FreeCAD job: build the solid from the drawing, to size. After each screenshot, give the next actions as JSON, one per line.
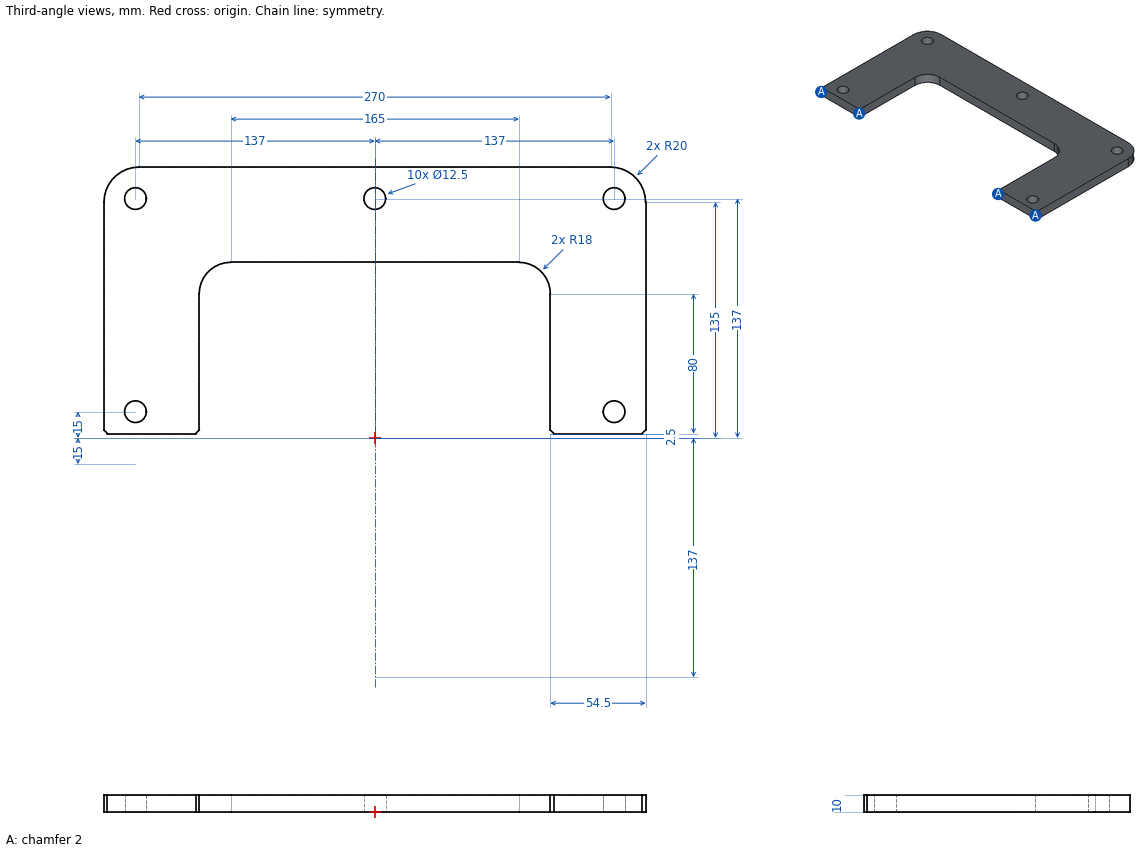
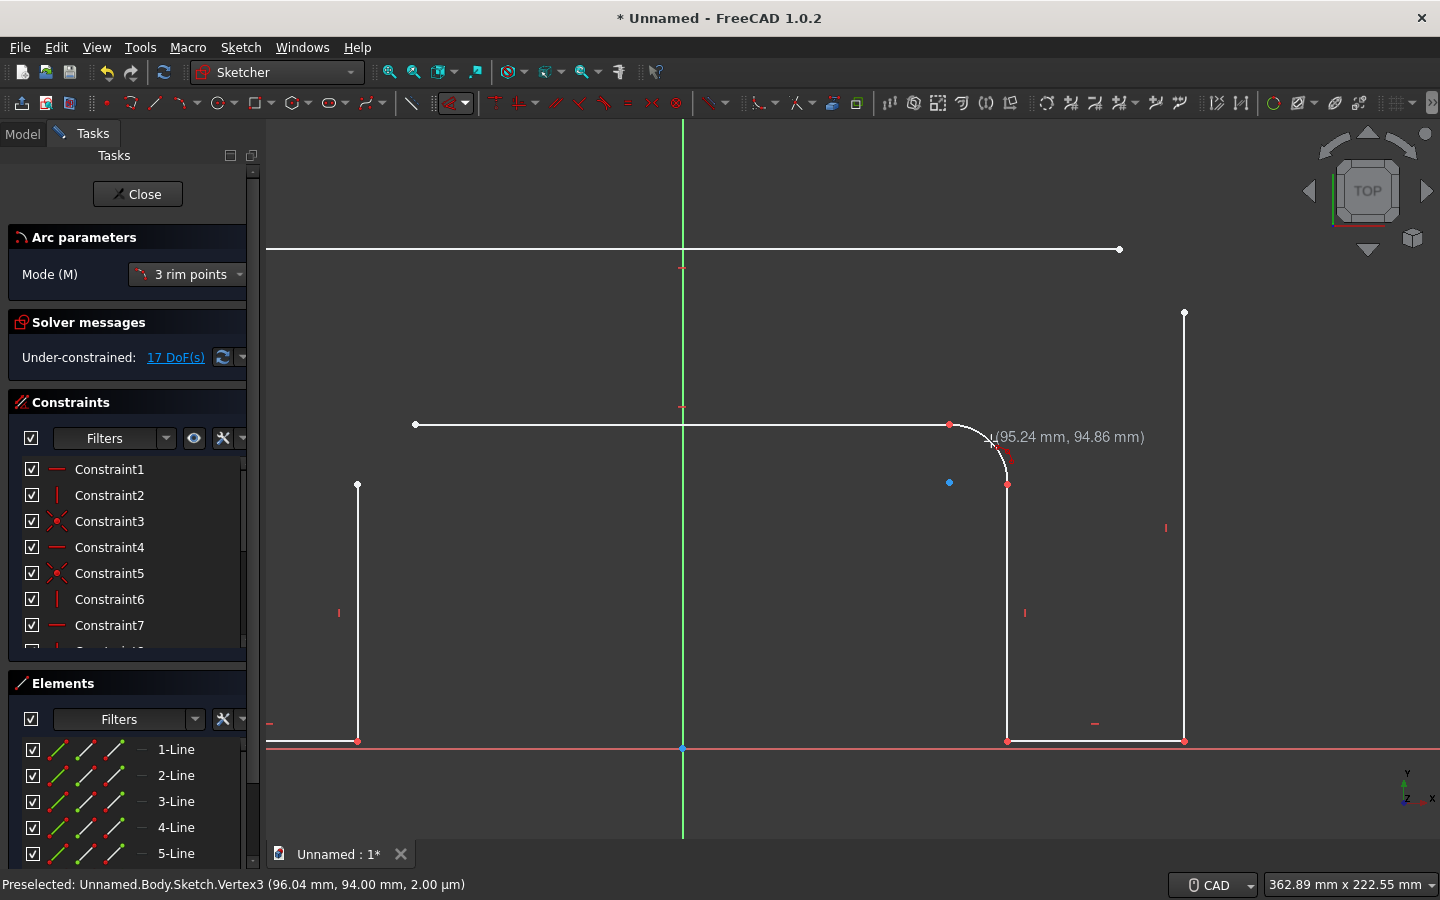
{"action": "left_click", "coordinate": [1184, 313]}
{"action": "left_click", "coordinate": [1119, 249]}
{"action": "left_click", "coordinate": [1165, 266]}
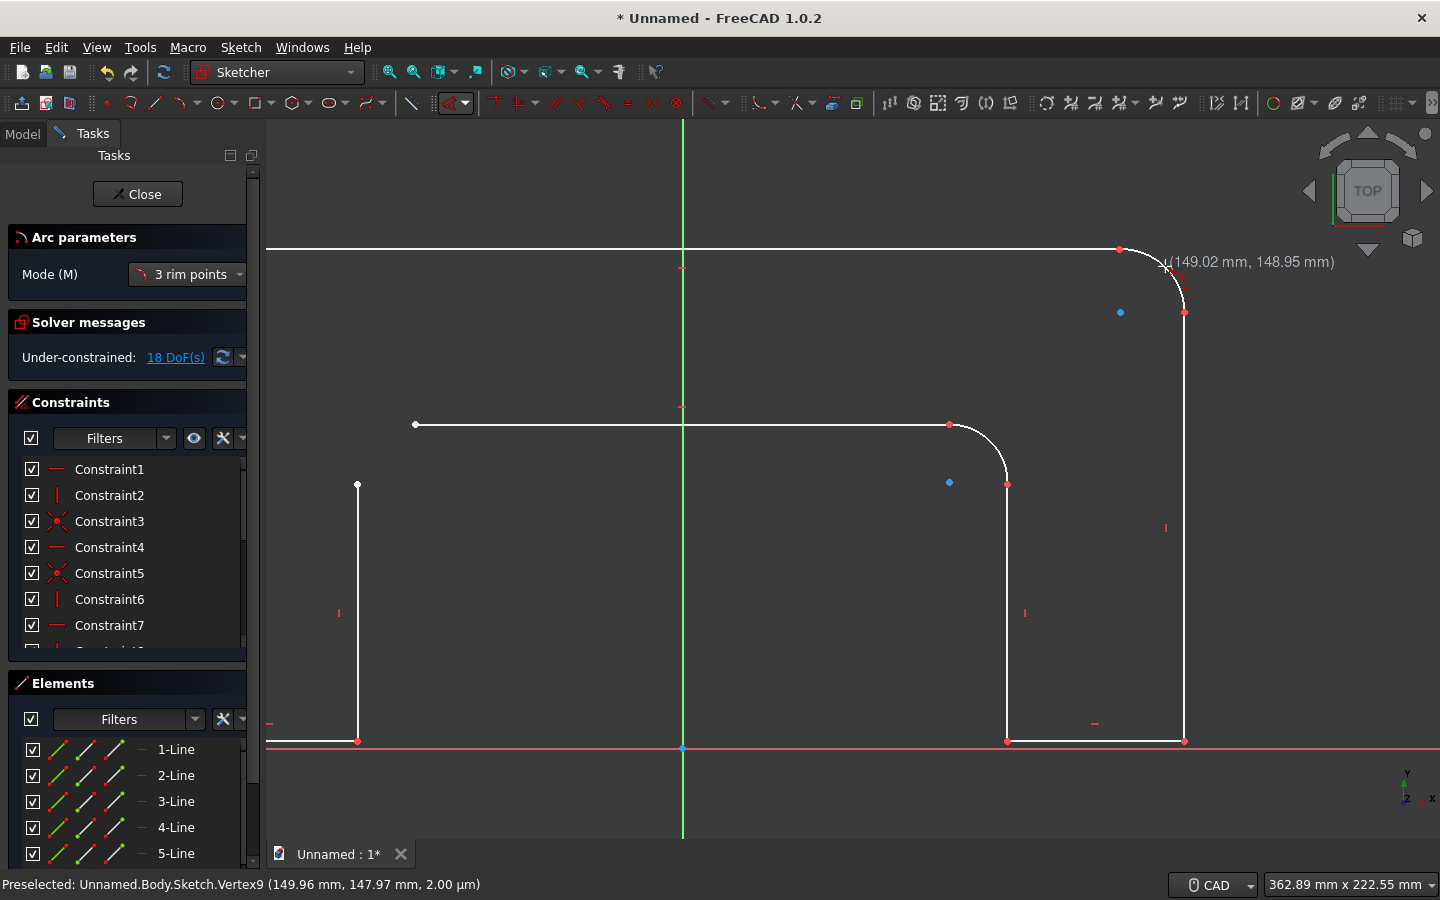
{"action": "scroll", "coordinate": [991, 440], "scroll_direction": "down", "scroll_amount": 2}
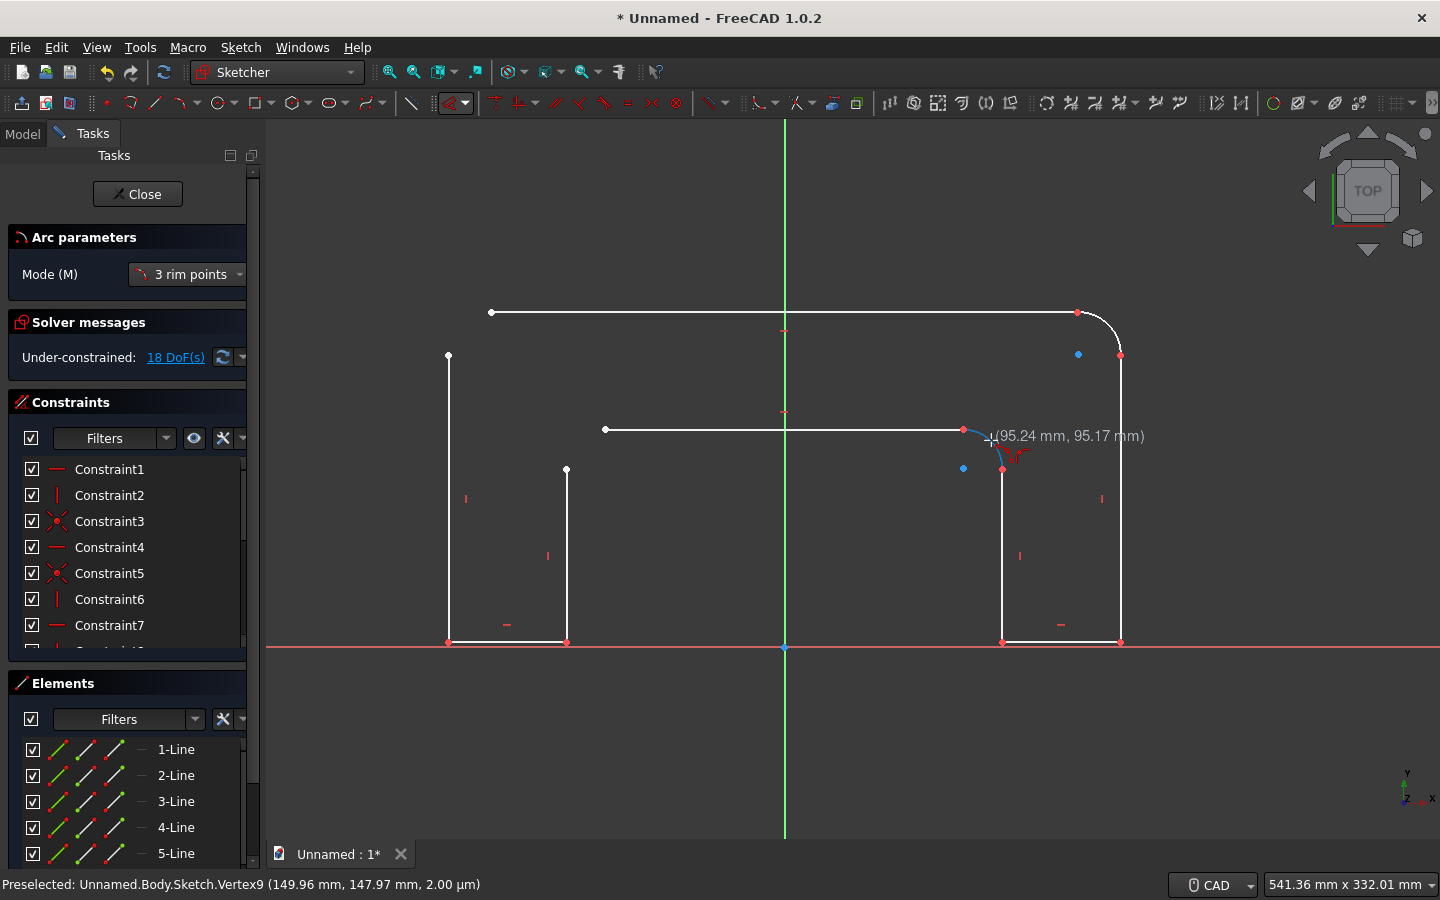
{"action": "left_click", "coordinate": [492, 312]}
{"action": "left_click", "coordinate": [449, 355]}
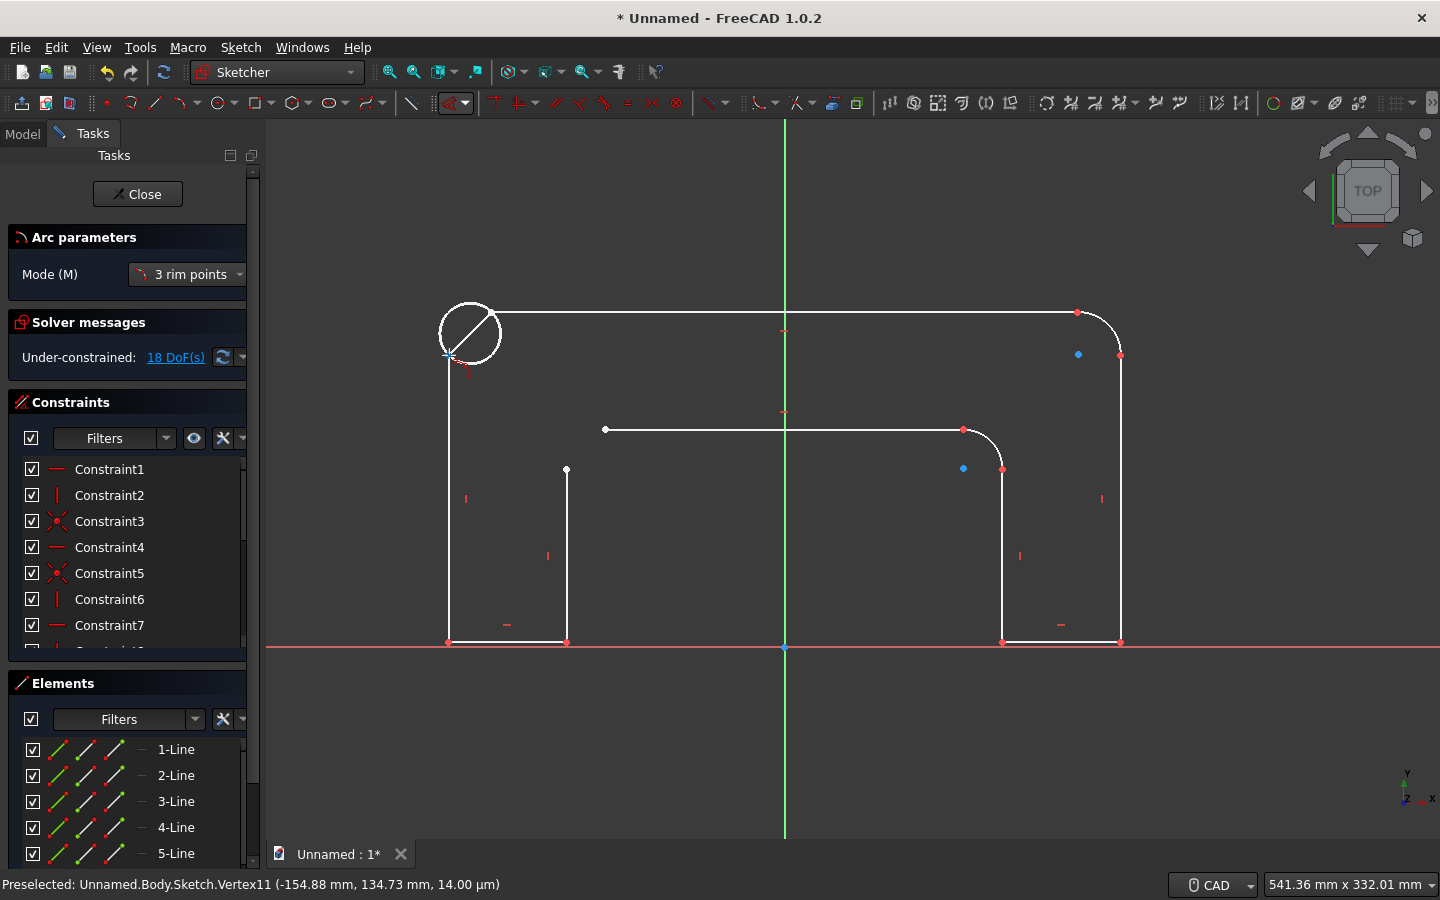
{"action": "scroll", "coordinate": [461, 324], "scroll_direction": "up", "scroll_amount": 2}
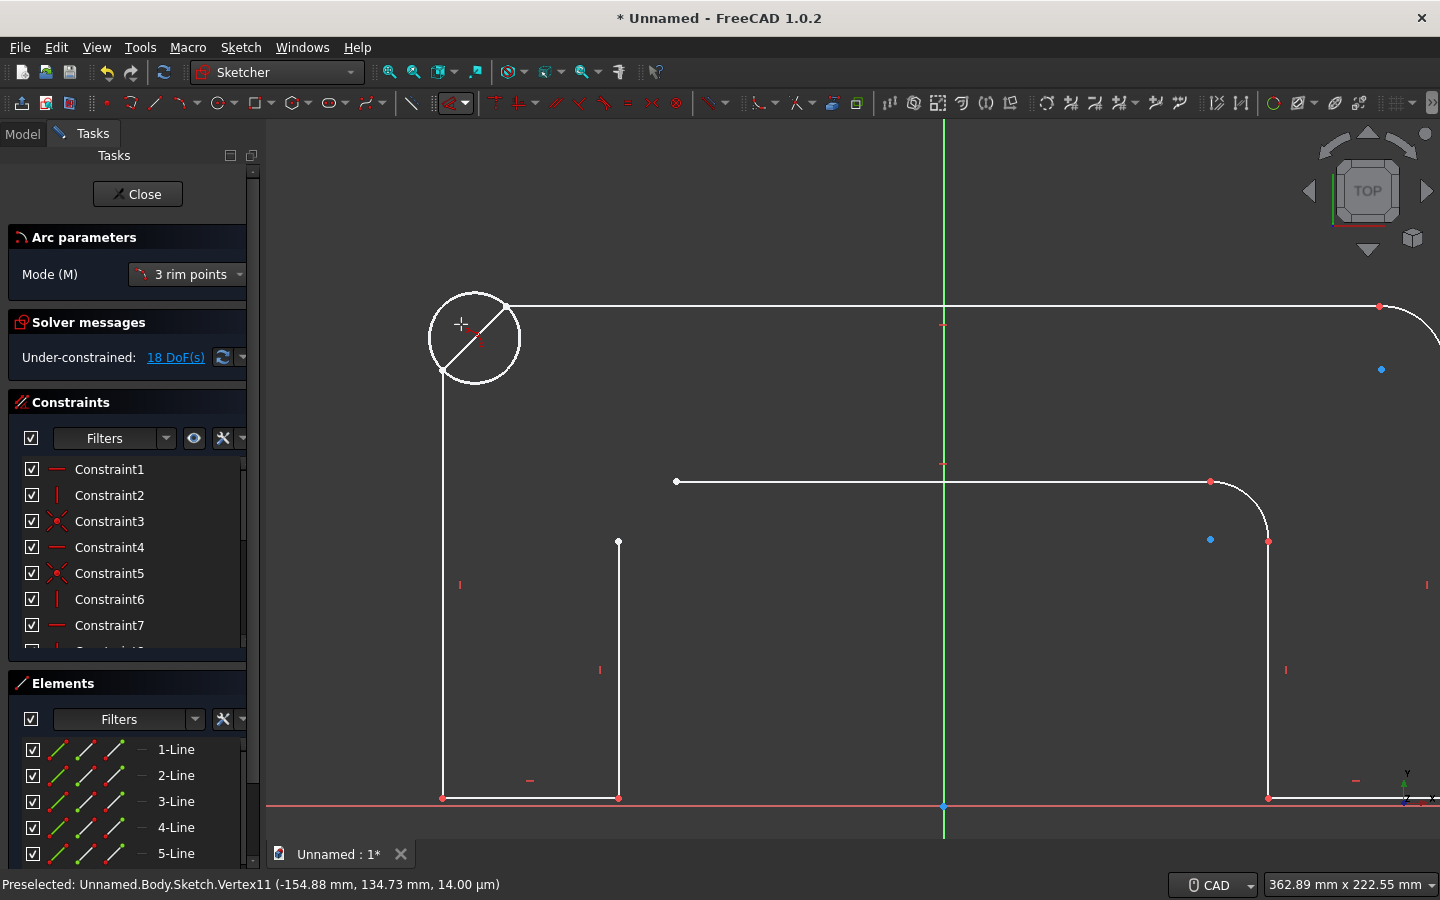
{"action": "left_click", "coordinate": [461, 324]}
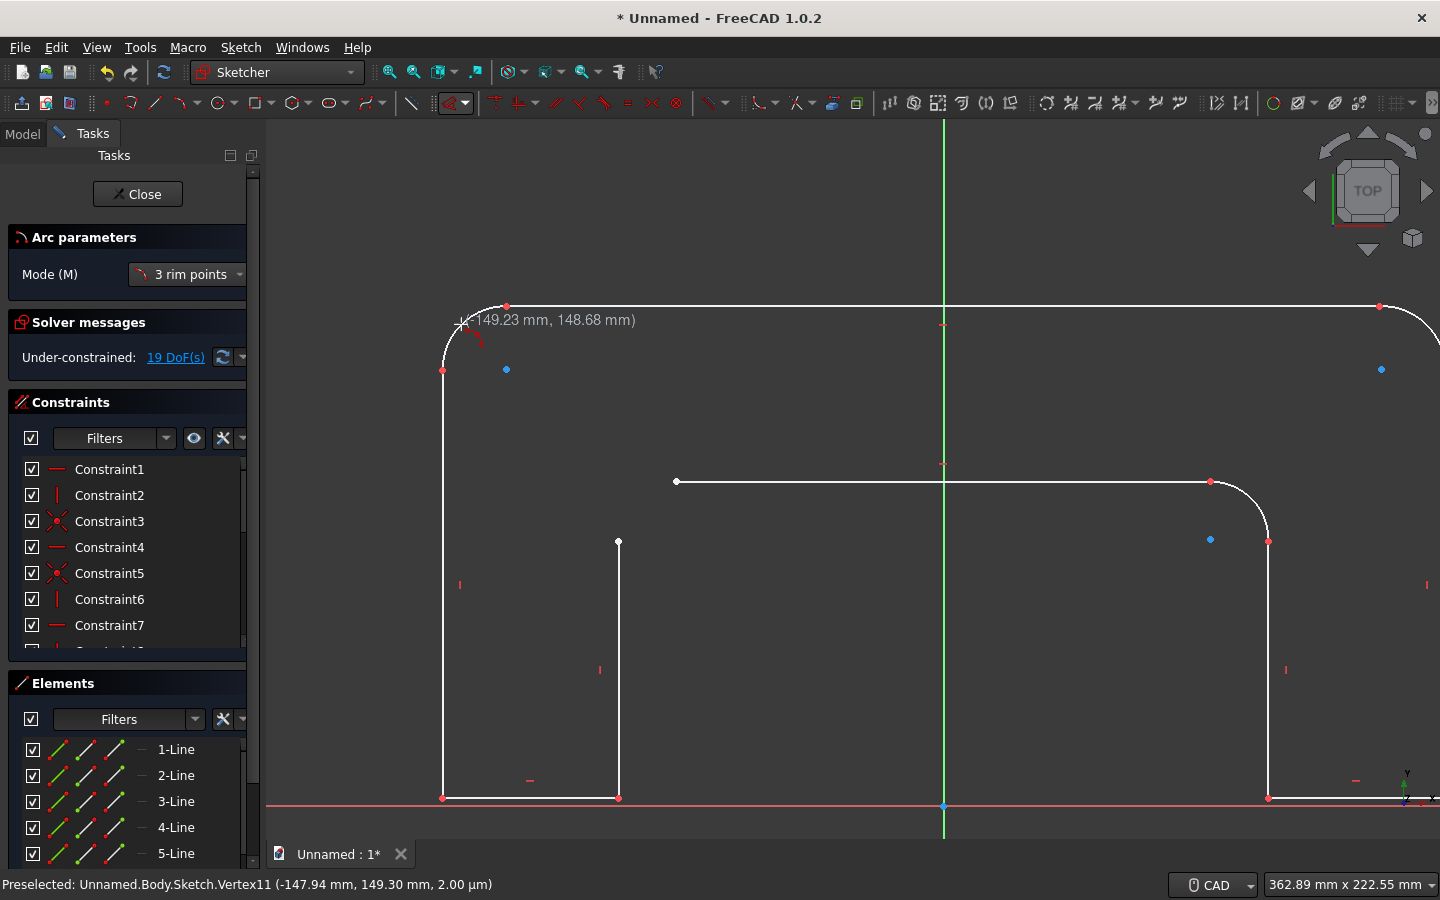
{"action": "left_click", "coordinate": [619, 541]}
{"action": "left_click", "coordinate": [676, 482]}
{"action": "left_click", "coordinate": [636, 498]}
{"action": "key", "text": "Escape"}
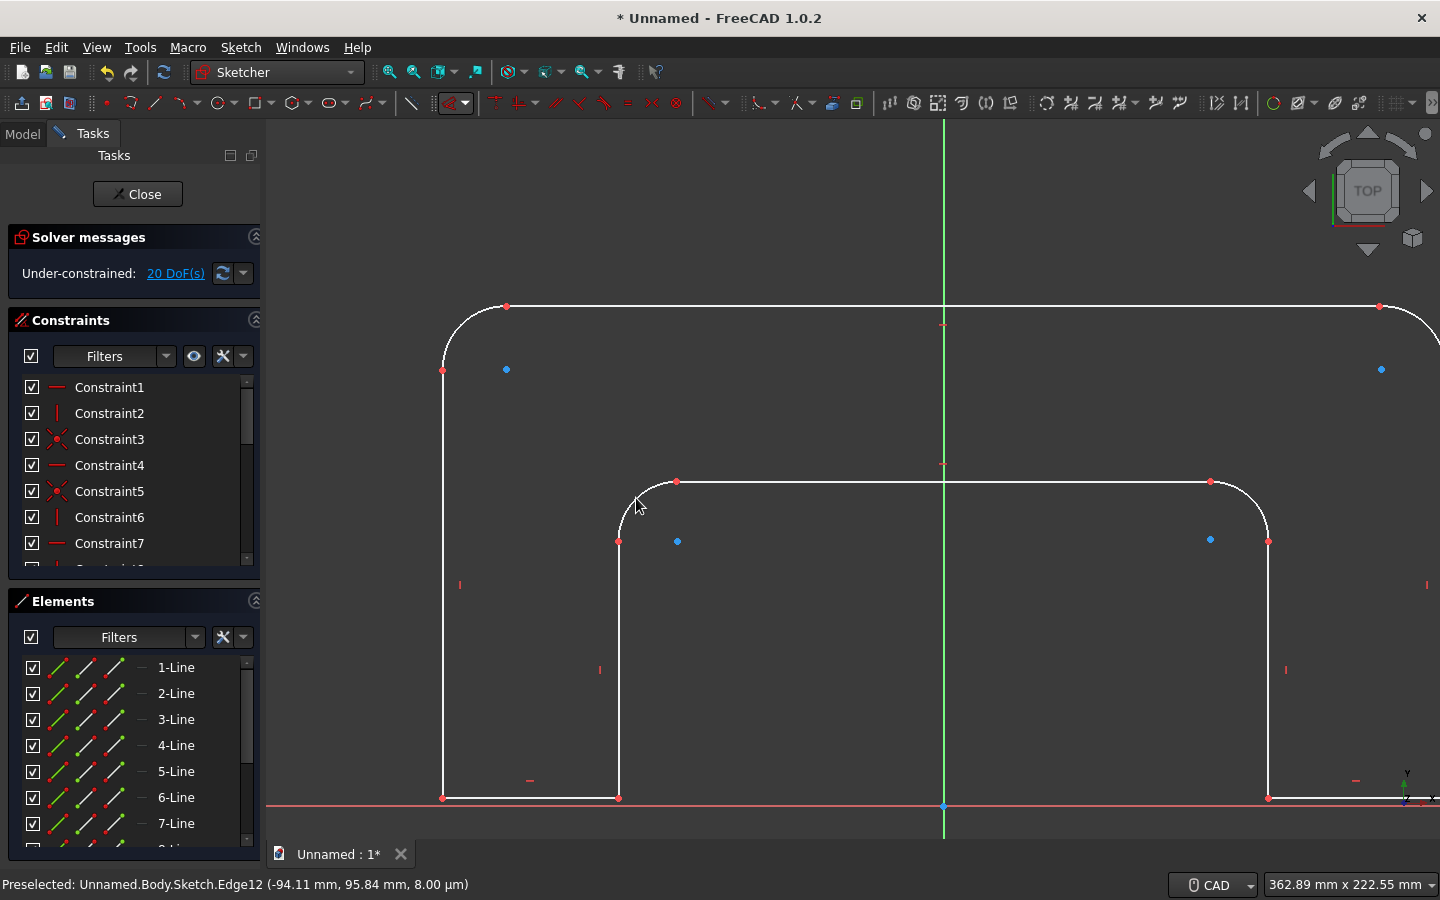
{"action": "left_click", "coordinate": [836, 482]}